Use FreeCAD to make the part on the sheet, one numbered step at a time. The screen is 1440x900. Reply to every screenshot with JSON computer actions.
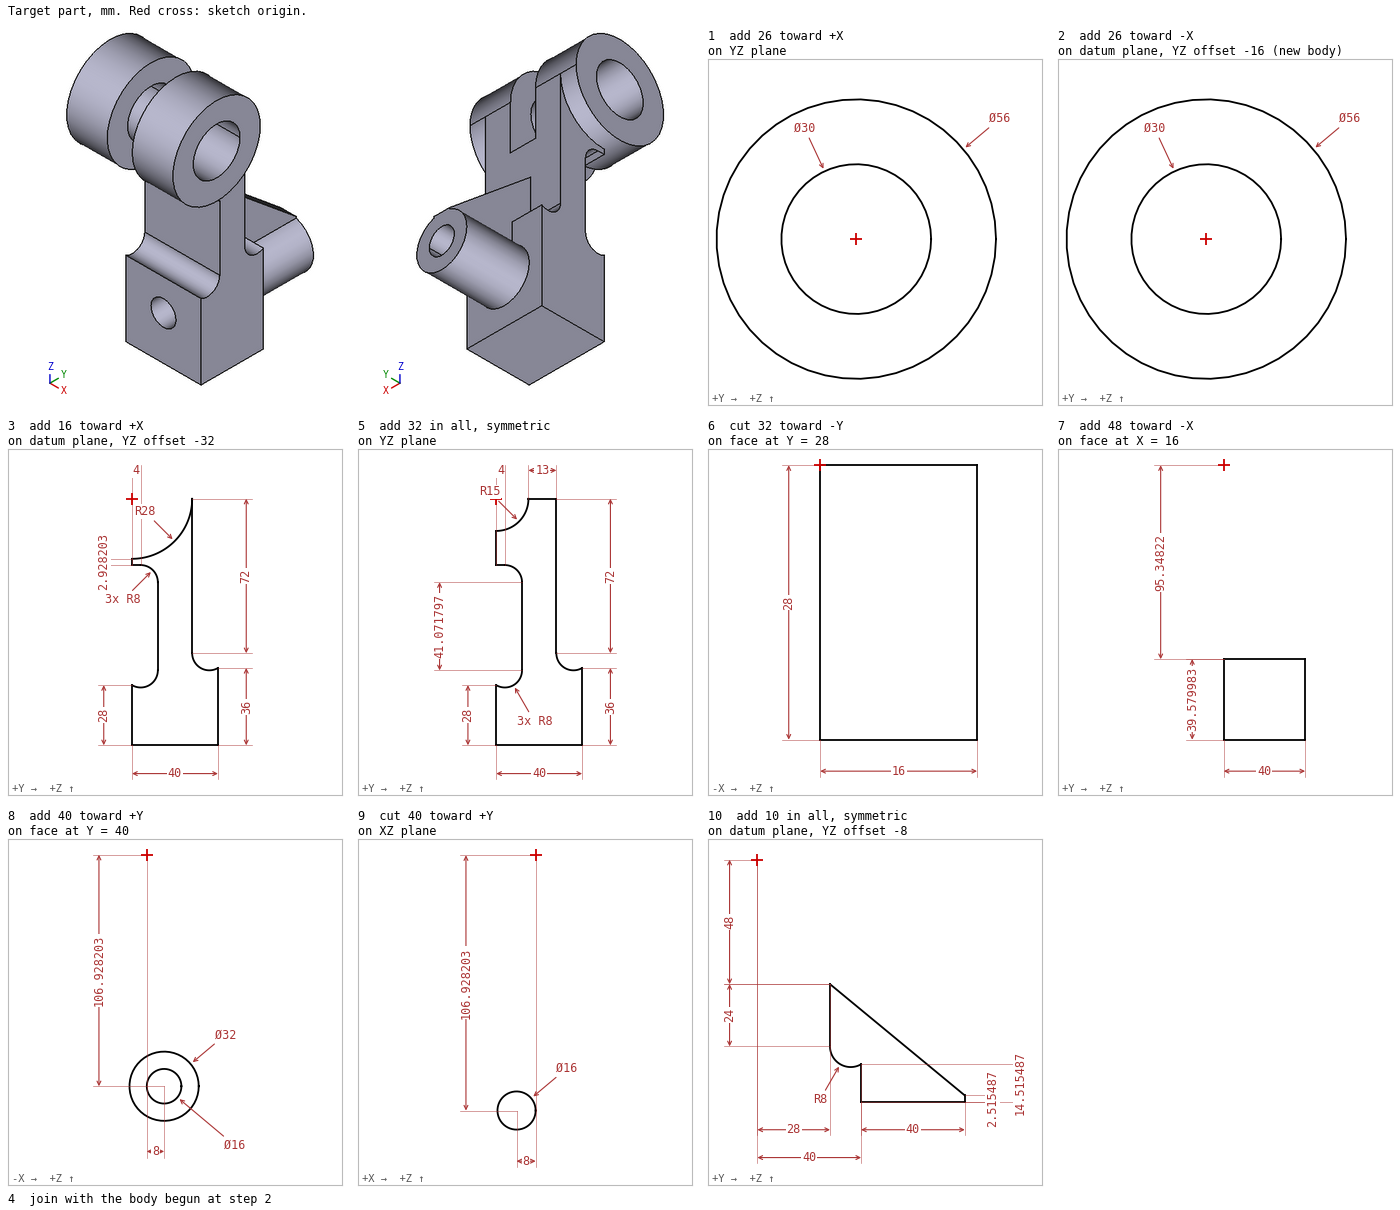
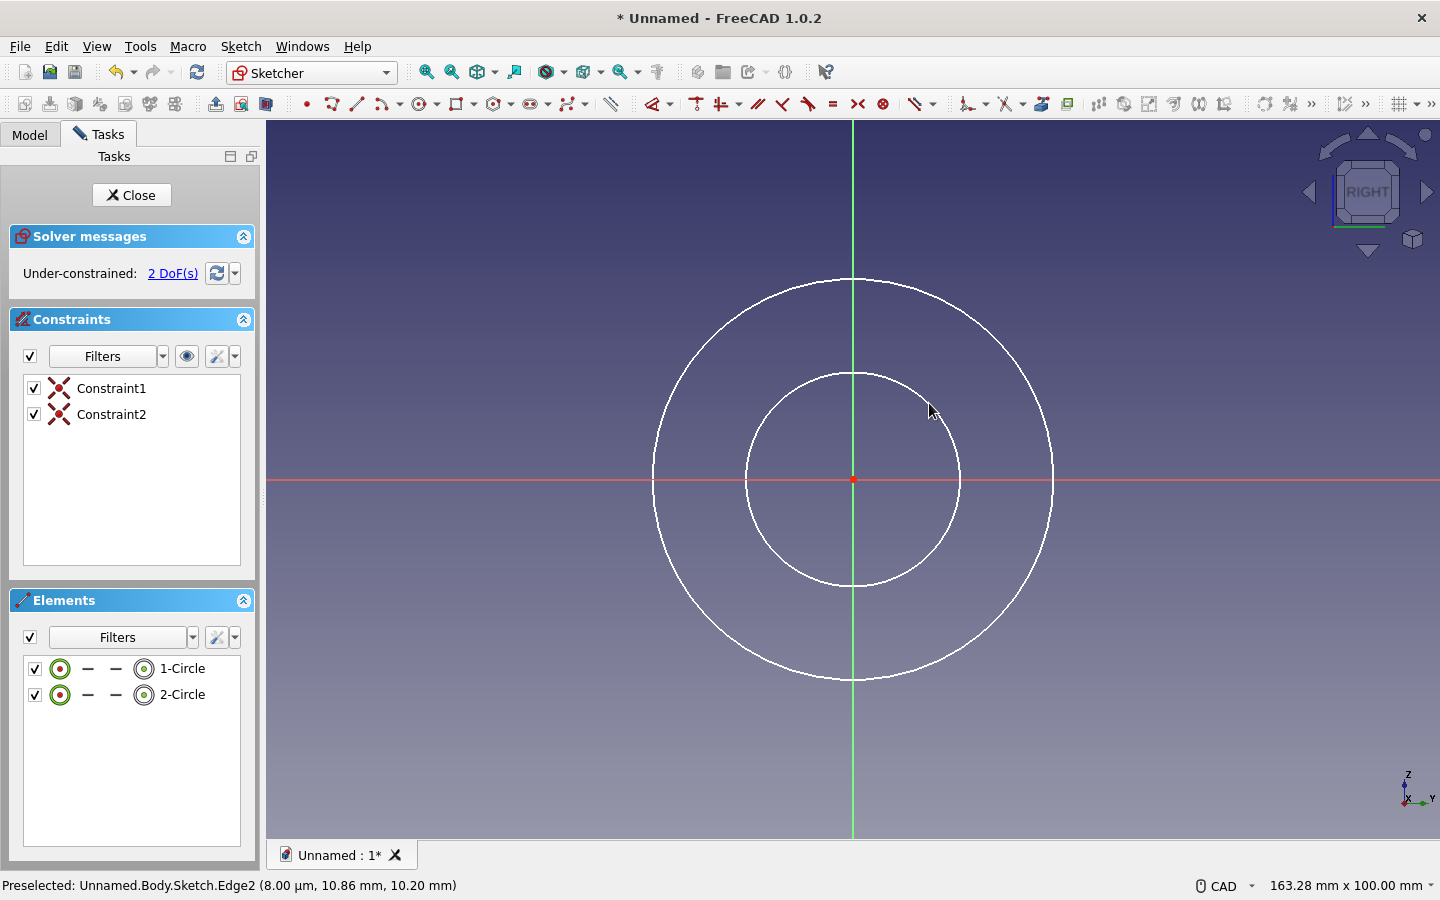
{"action": "left_click", "coordinate": [652, 104]}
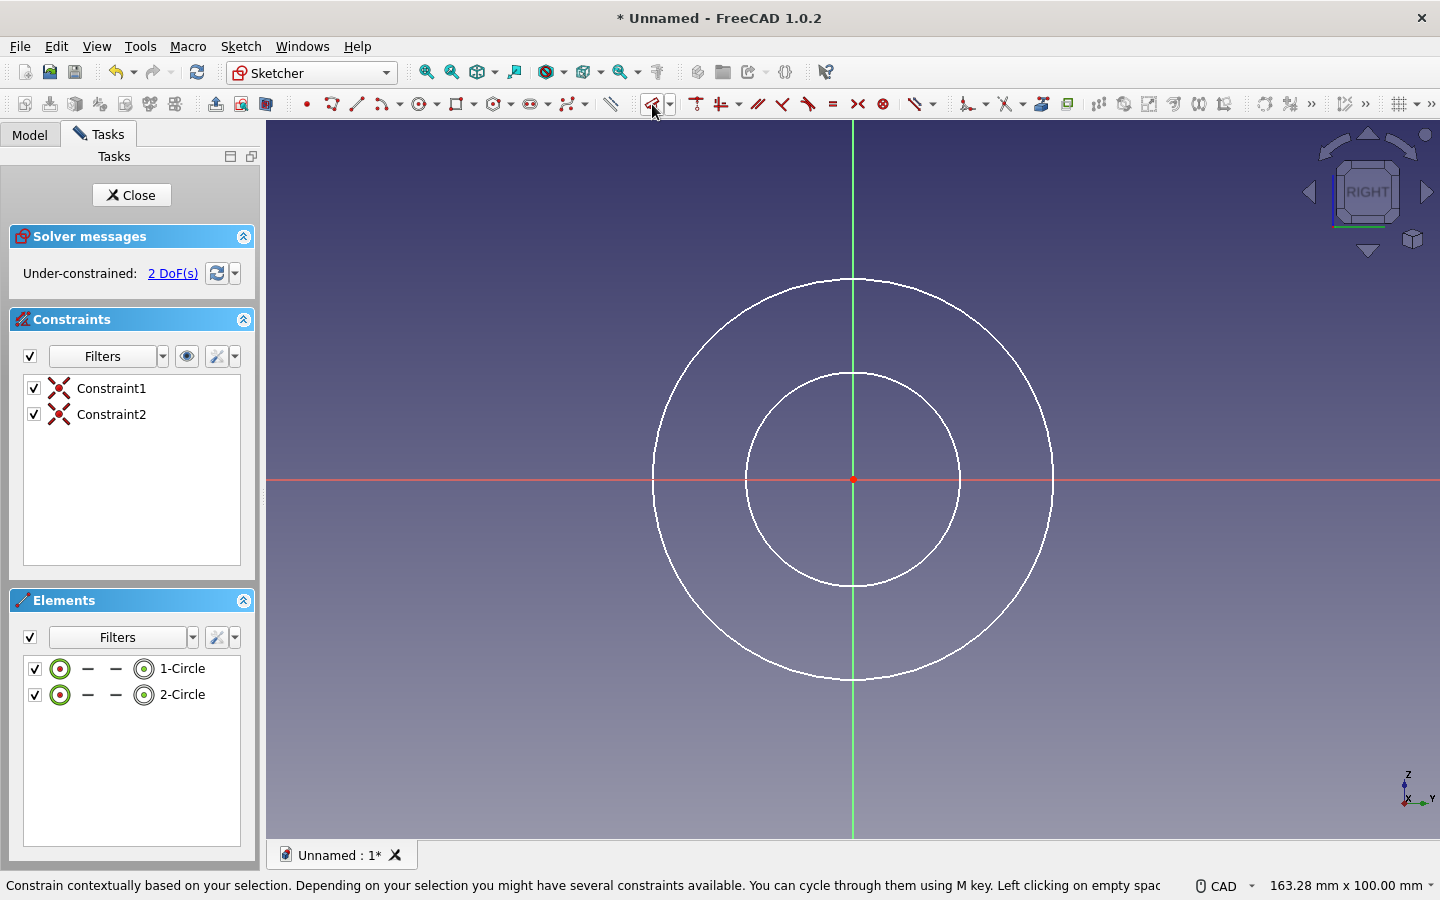
{"action": "left_click", "coordinate": [994, 337]}
{"action": "left_click", "coordinate": [1017, 314]}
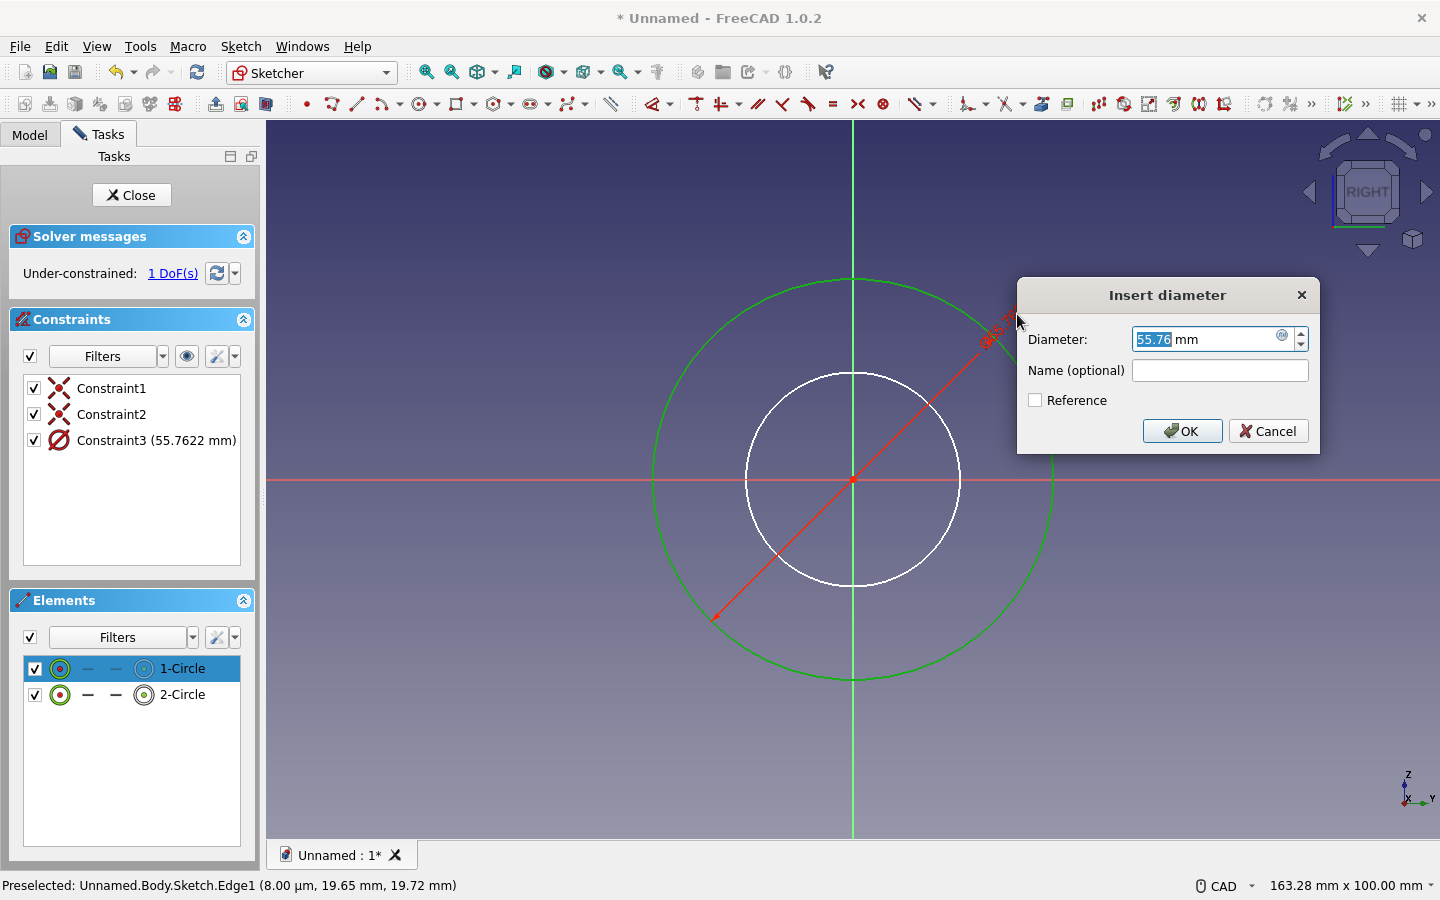
{"action": "type", "text": "56"}
{"action": "key", "text": "Return"}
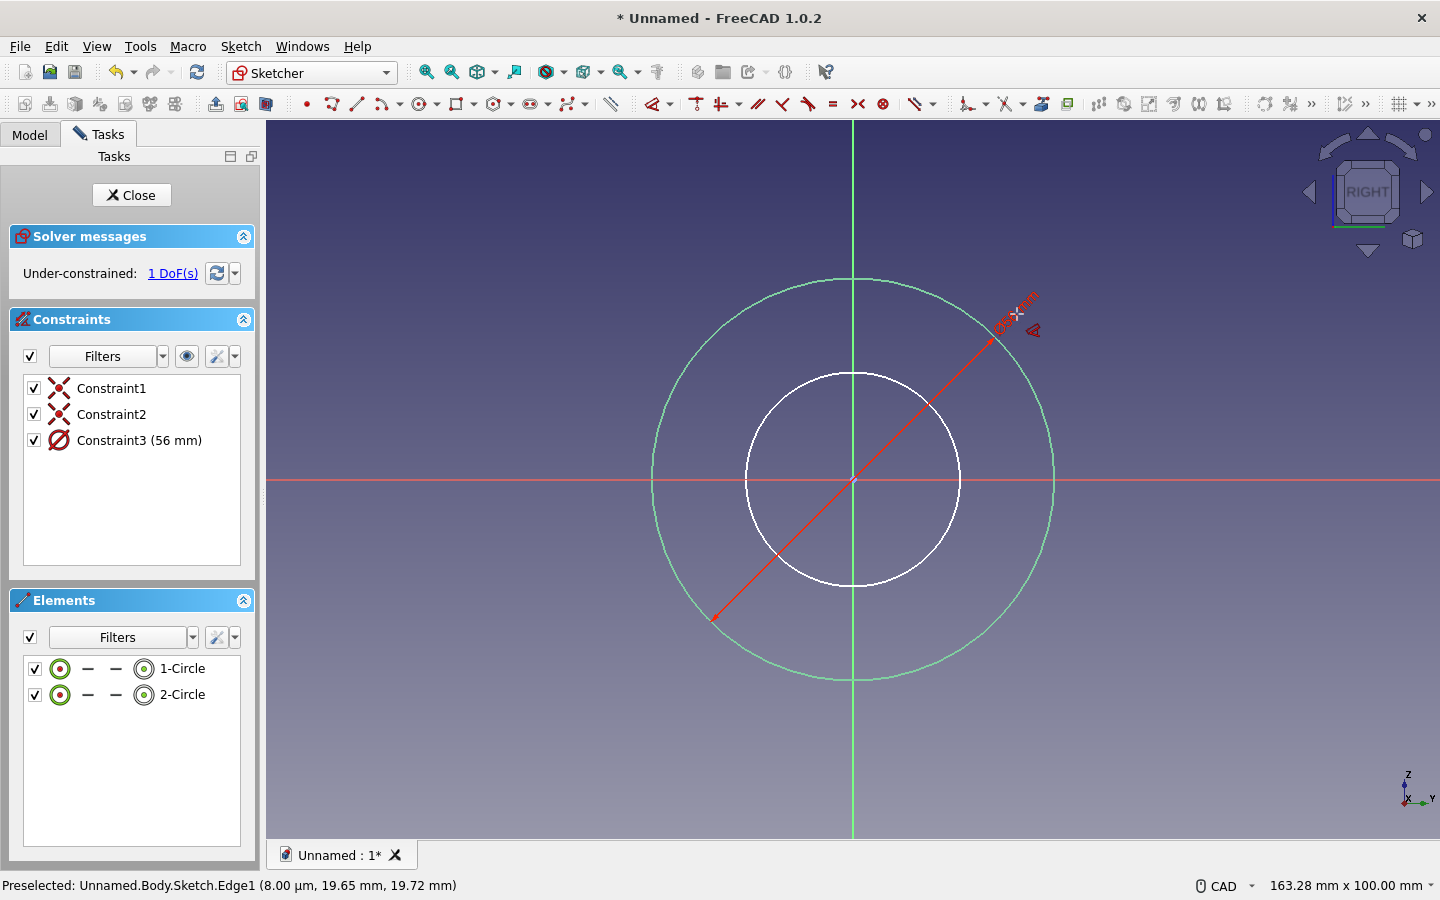
{"action": "left_click", "coordinate": [929, 404]}
{"action": "left_click", "coordinate": [952, 381]}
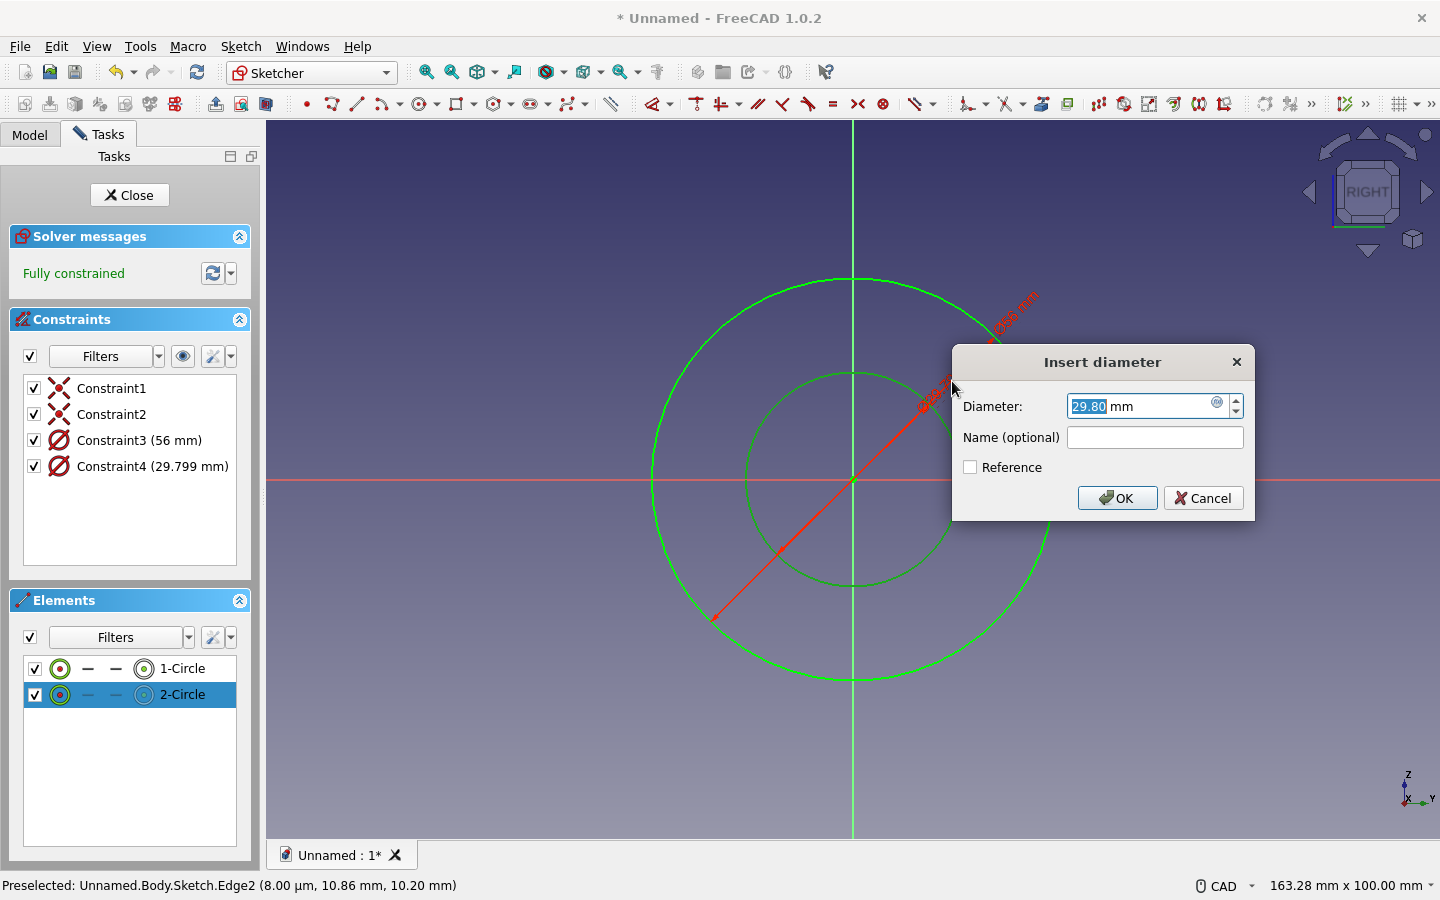
{"action": "type", "text": "30"}
{"action": "key", "text": "Return"}
{"action": "key", "text": "Escape"}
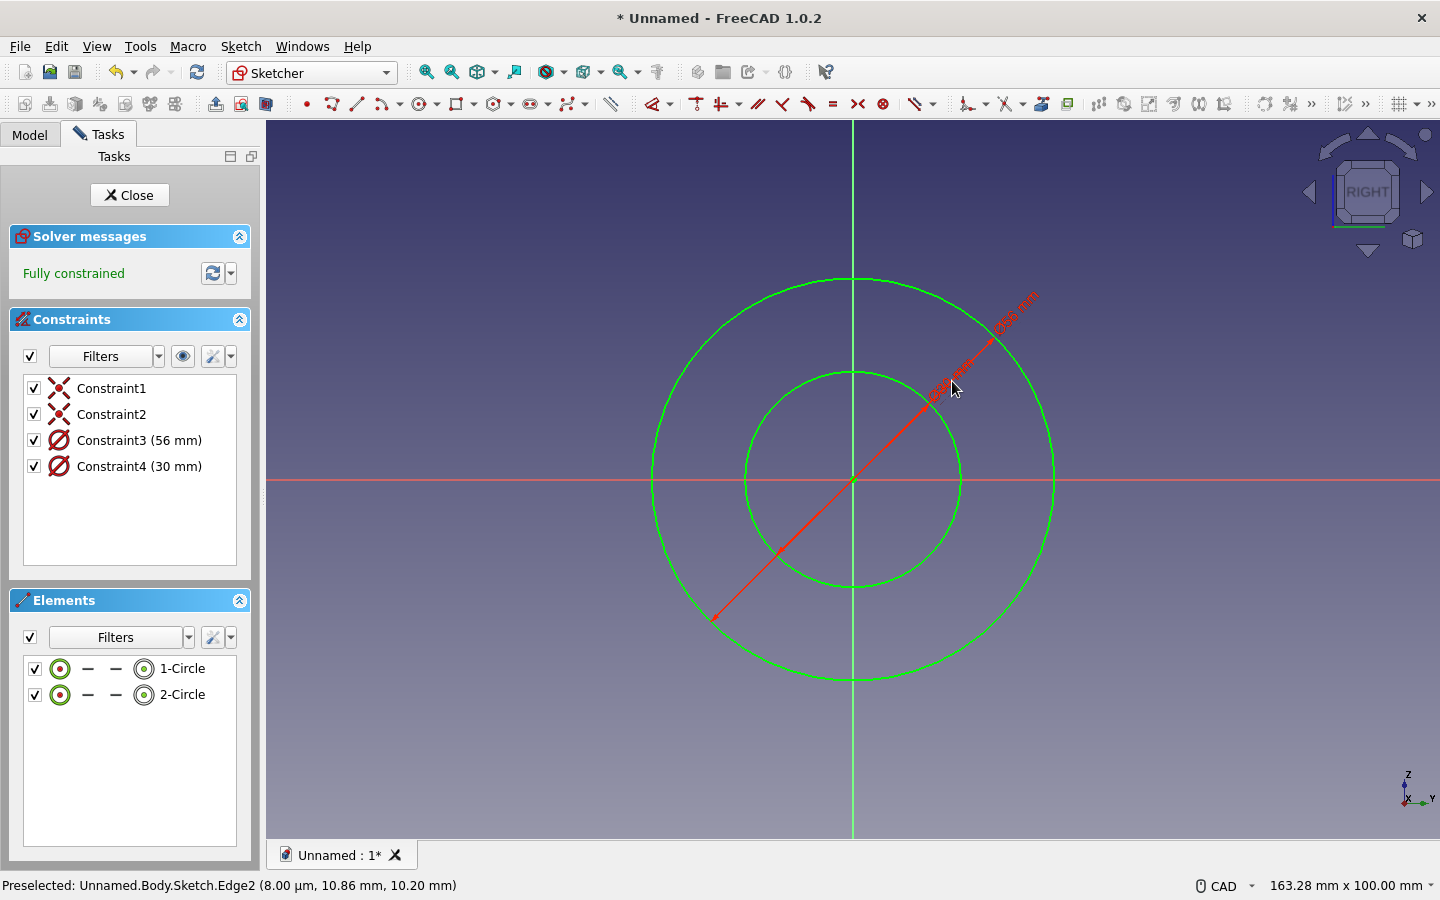
{"action": "left_click", "coordinate": [130, 195]}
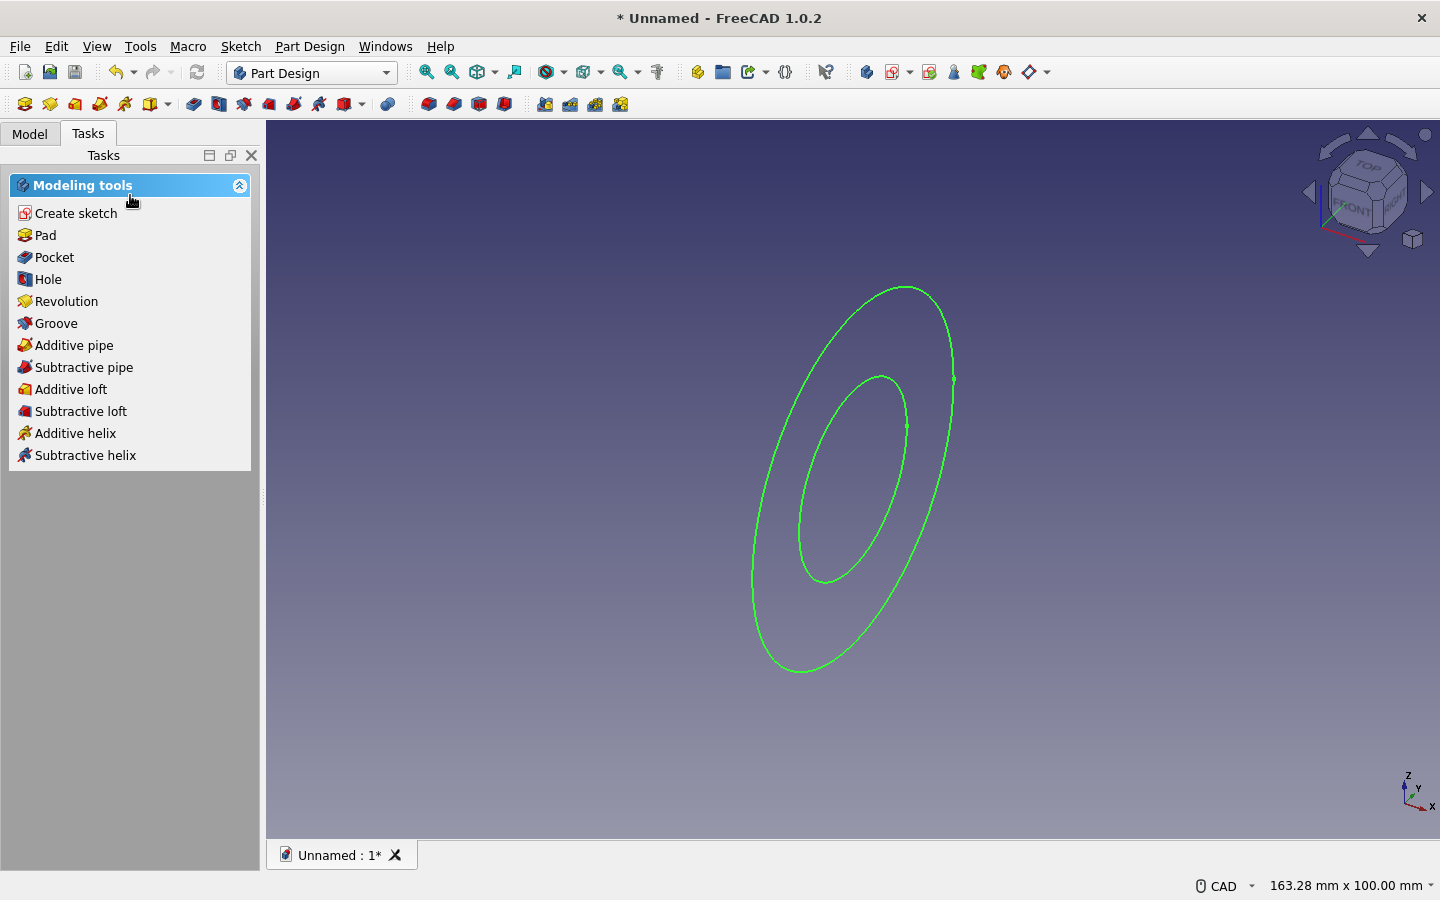
{"action": "left_click", "coordinate": [25, 104]}